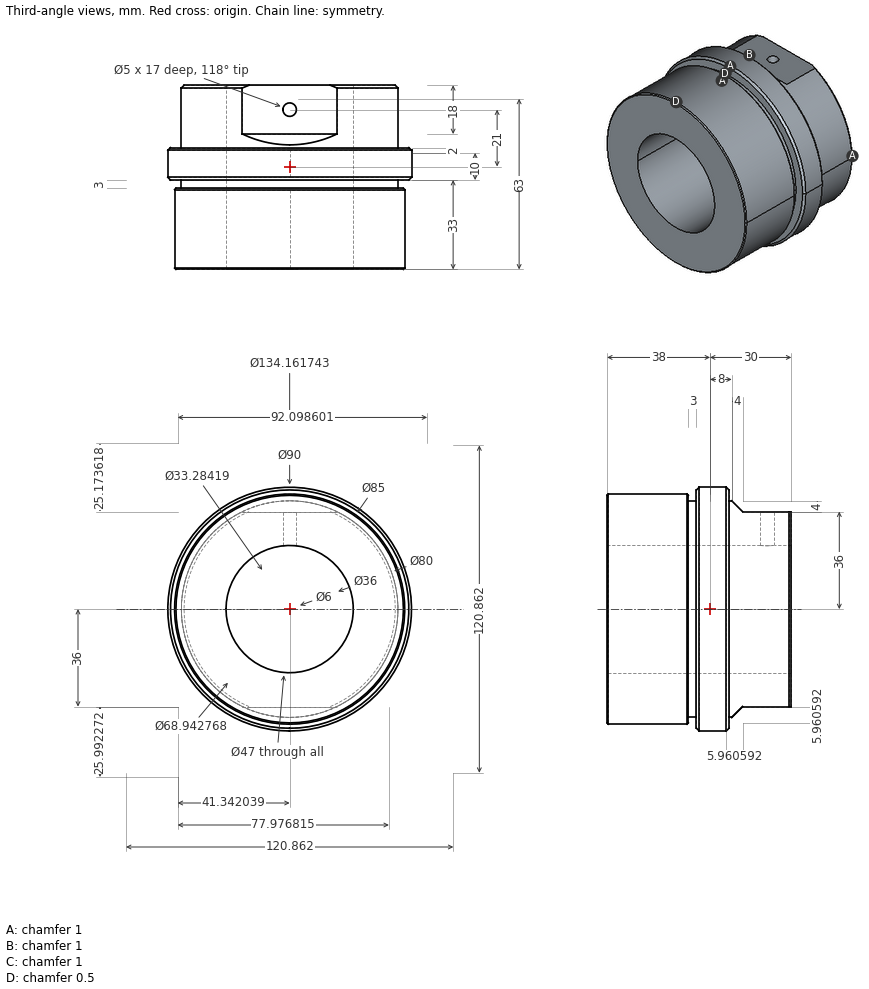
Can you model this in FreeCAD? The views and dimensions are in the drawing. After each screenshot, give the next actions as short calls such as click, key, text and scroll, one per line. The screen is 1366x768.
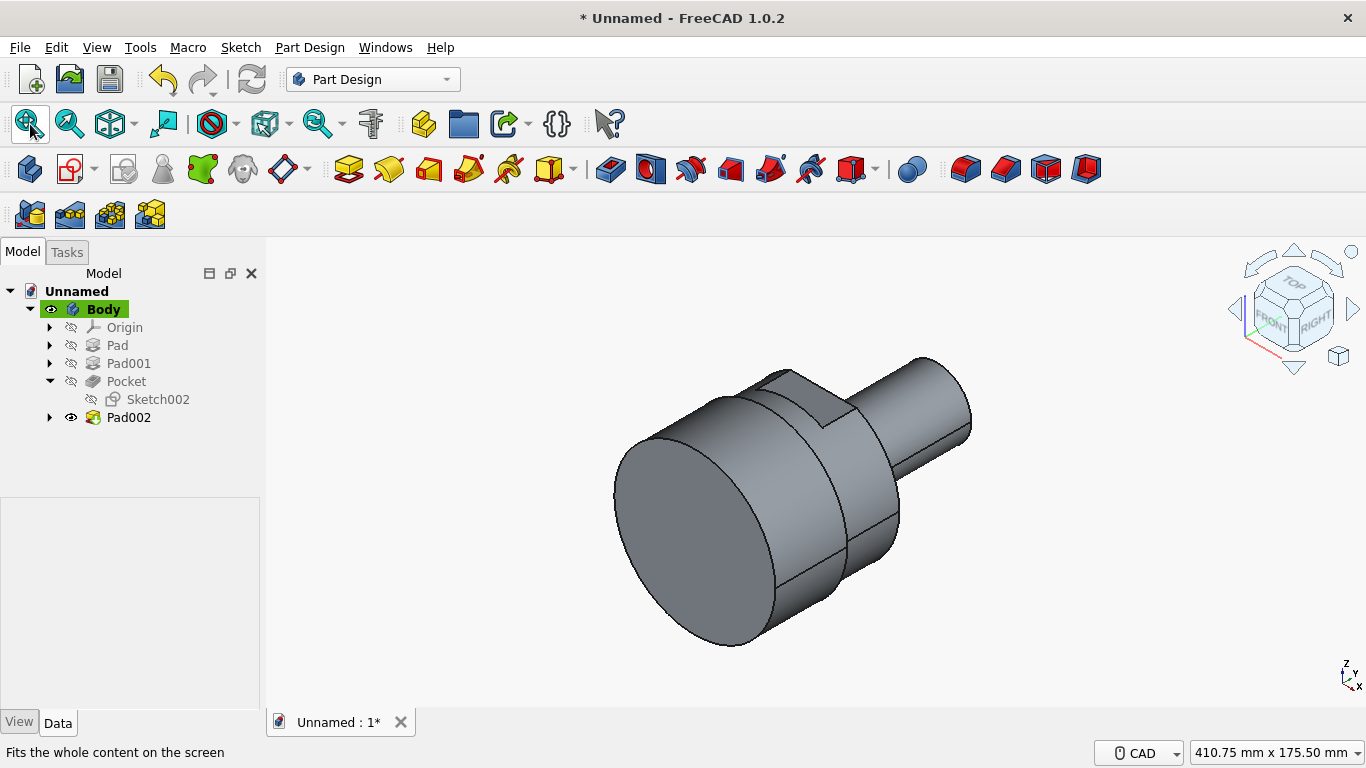
click(695, 541)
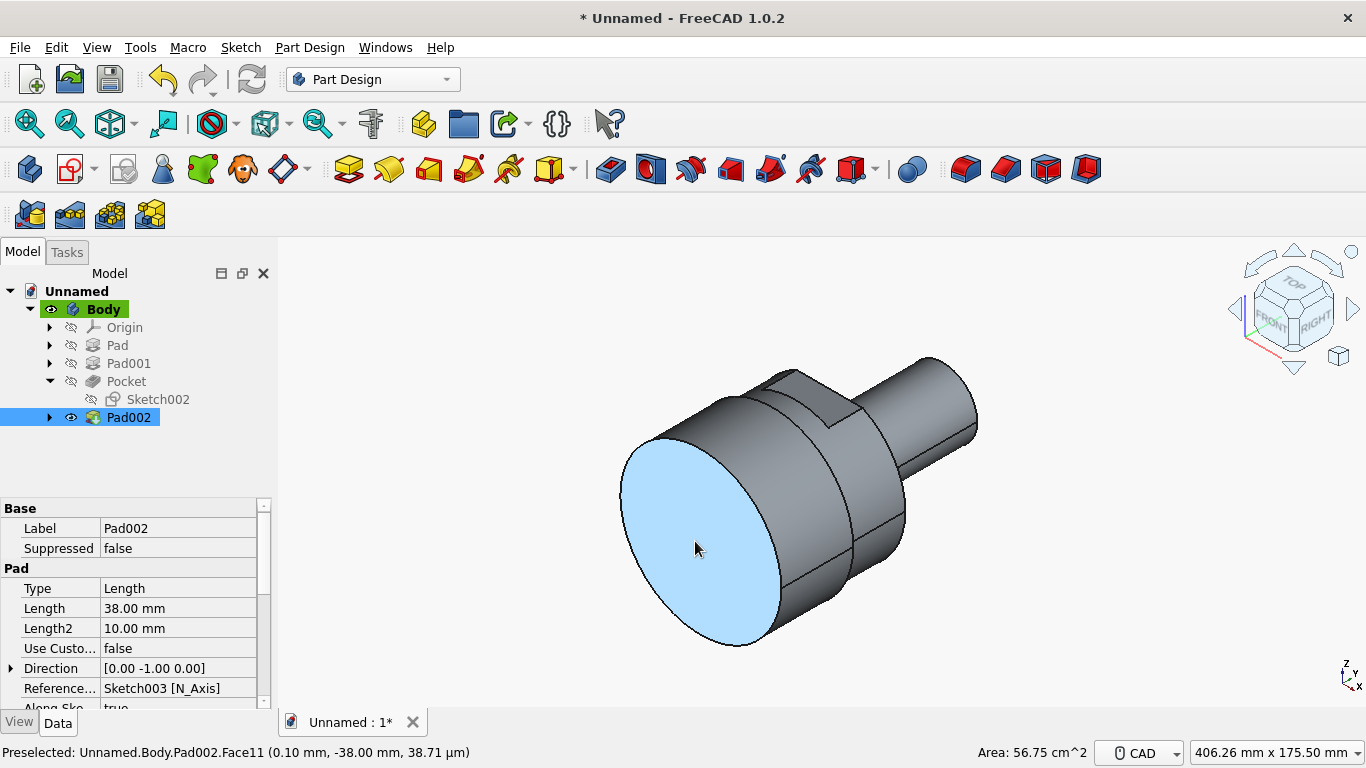
click(70, 170)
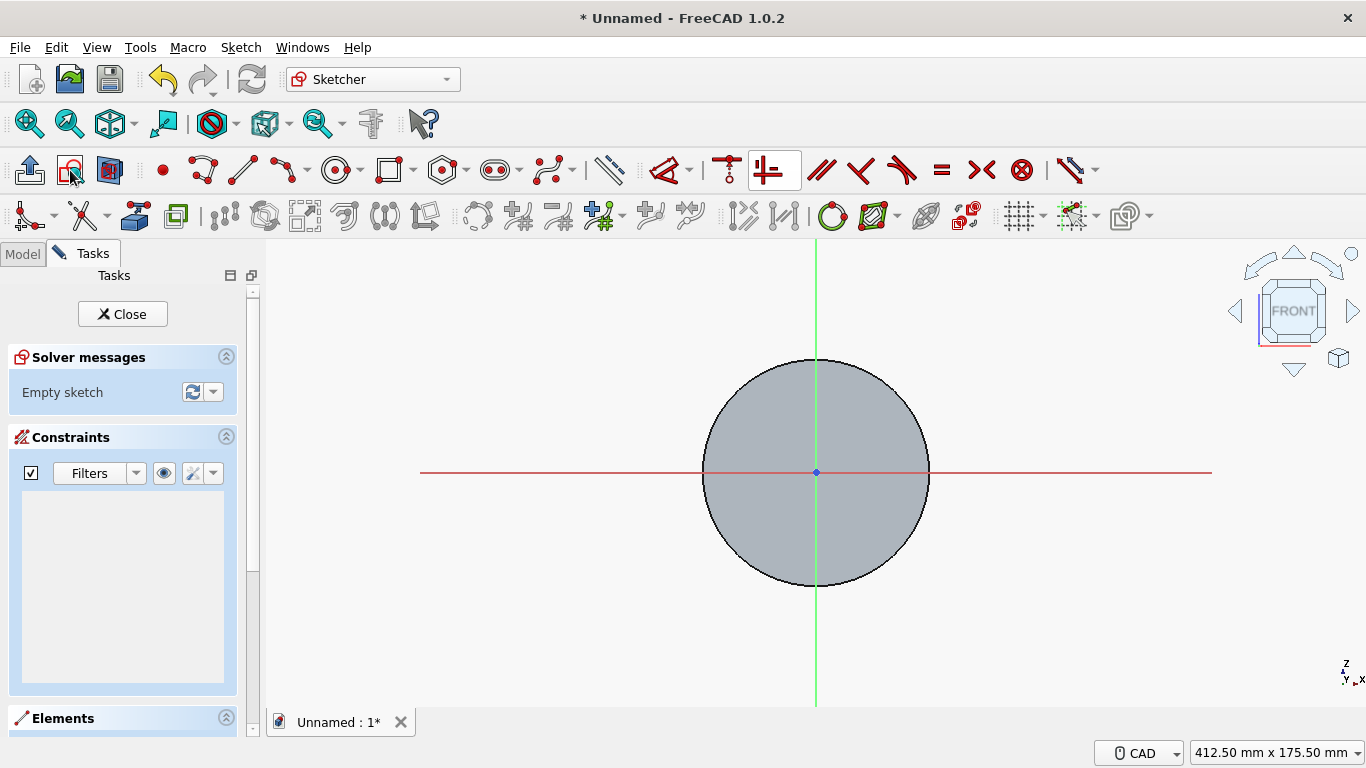
scroll(820, 473, up, 14)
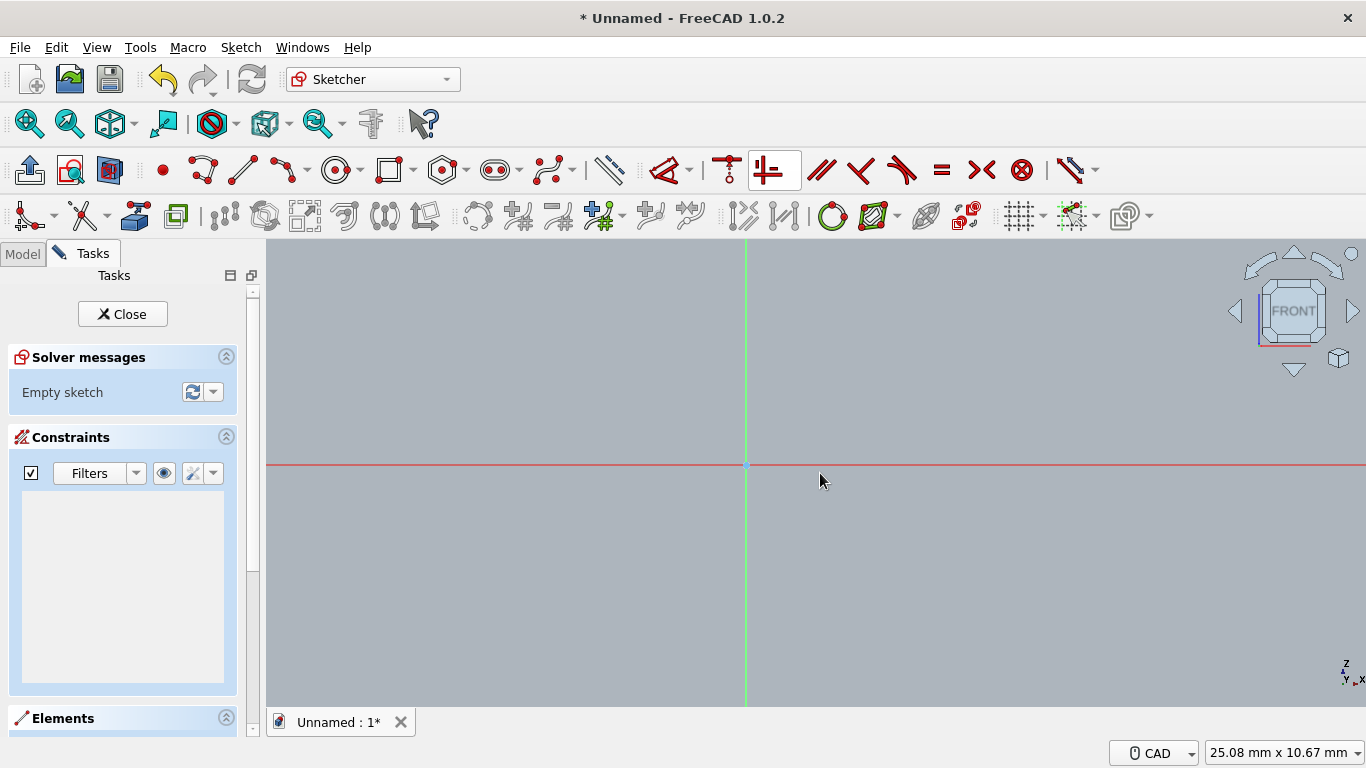
click(336, 170)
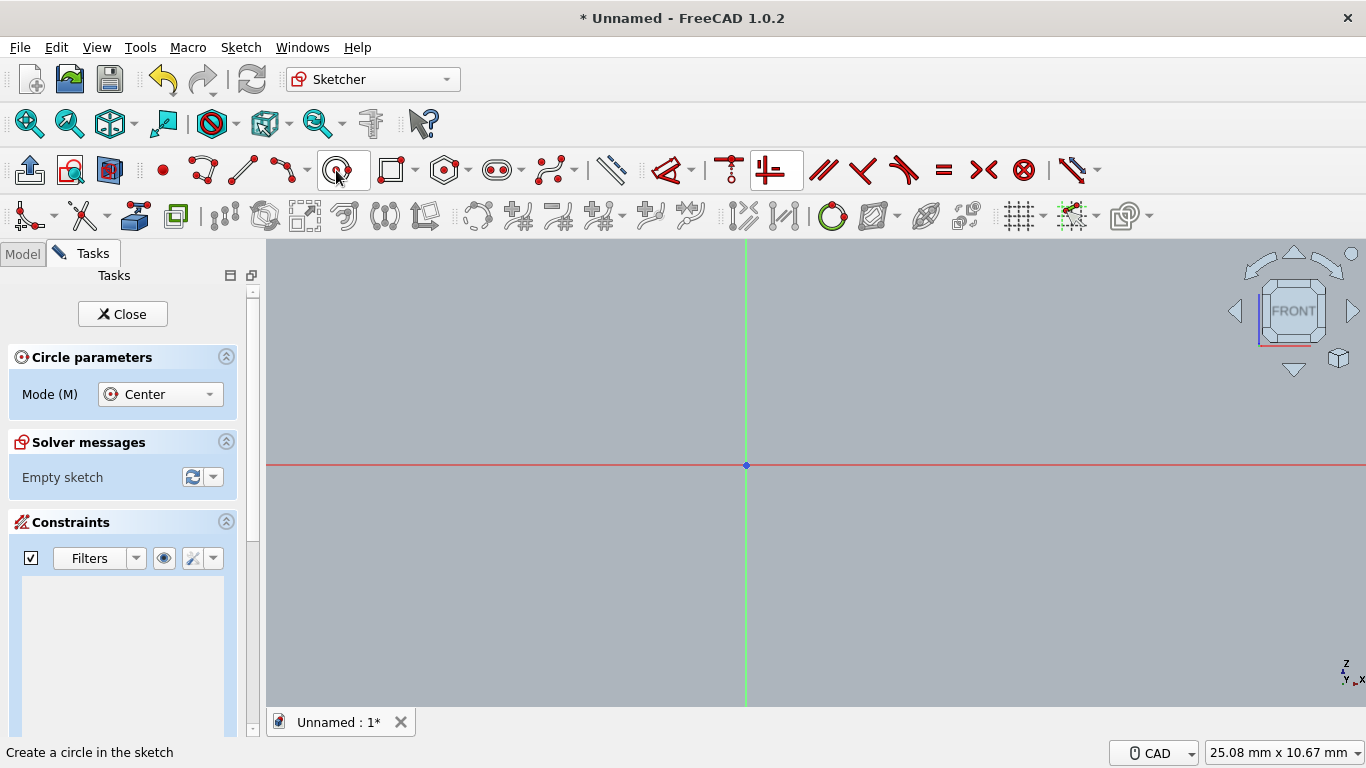
click(746, 465)
click(839, 372)
key(Escape)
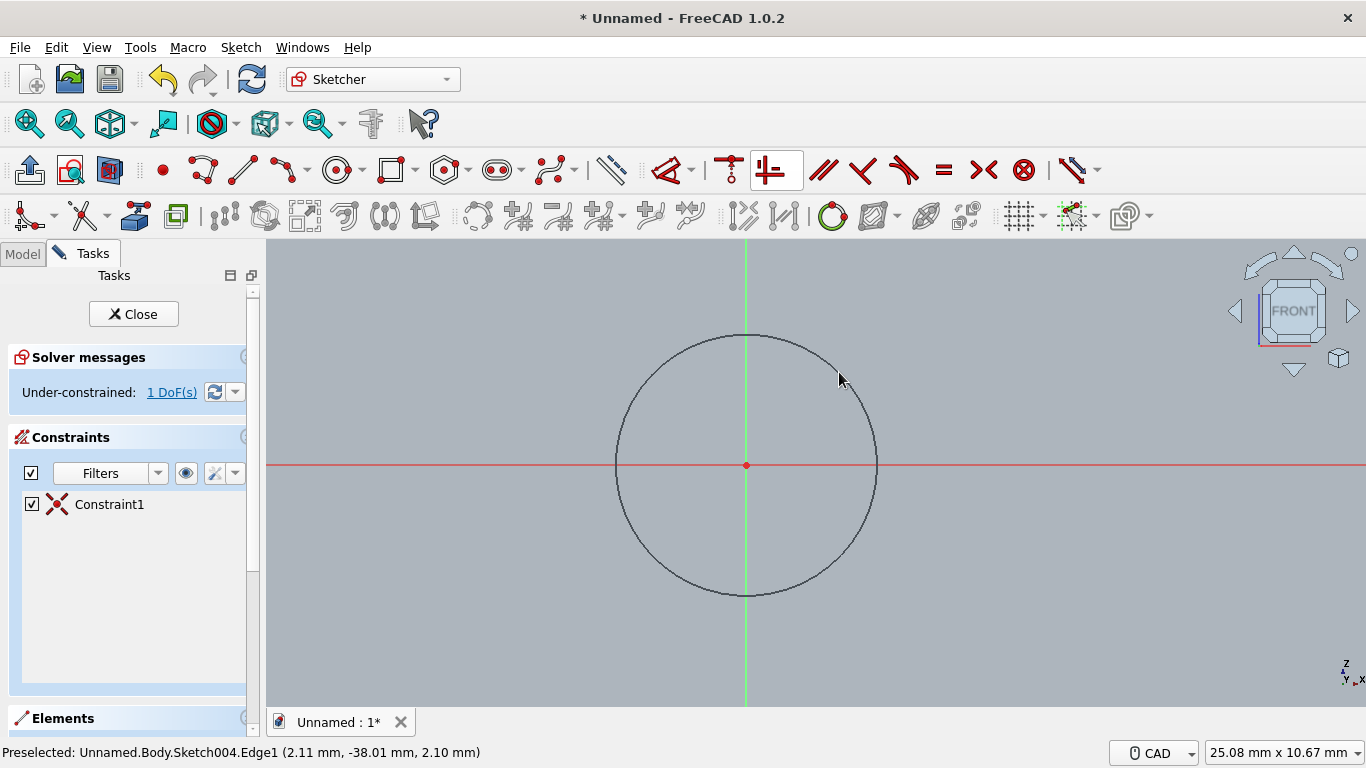
click(666, 170)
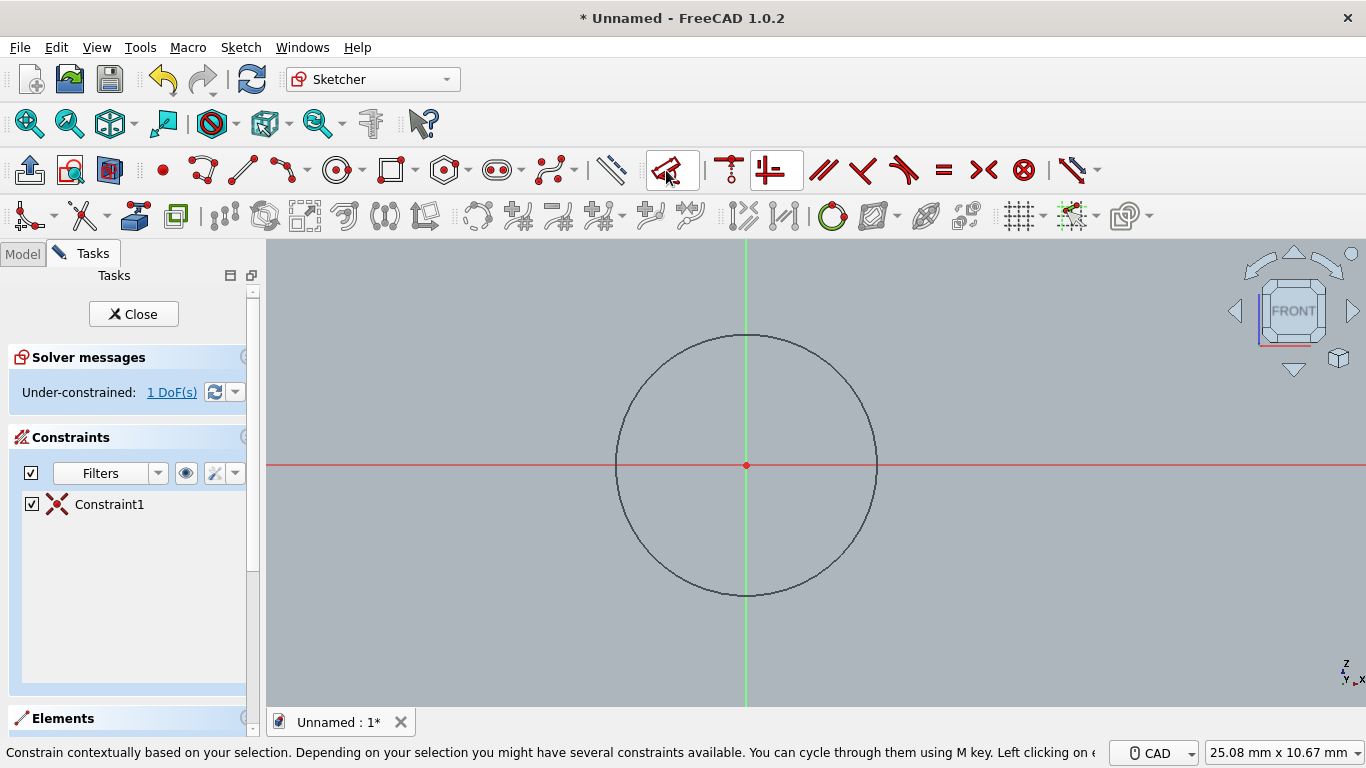
click(839, 373)
click(862, 350)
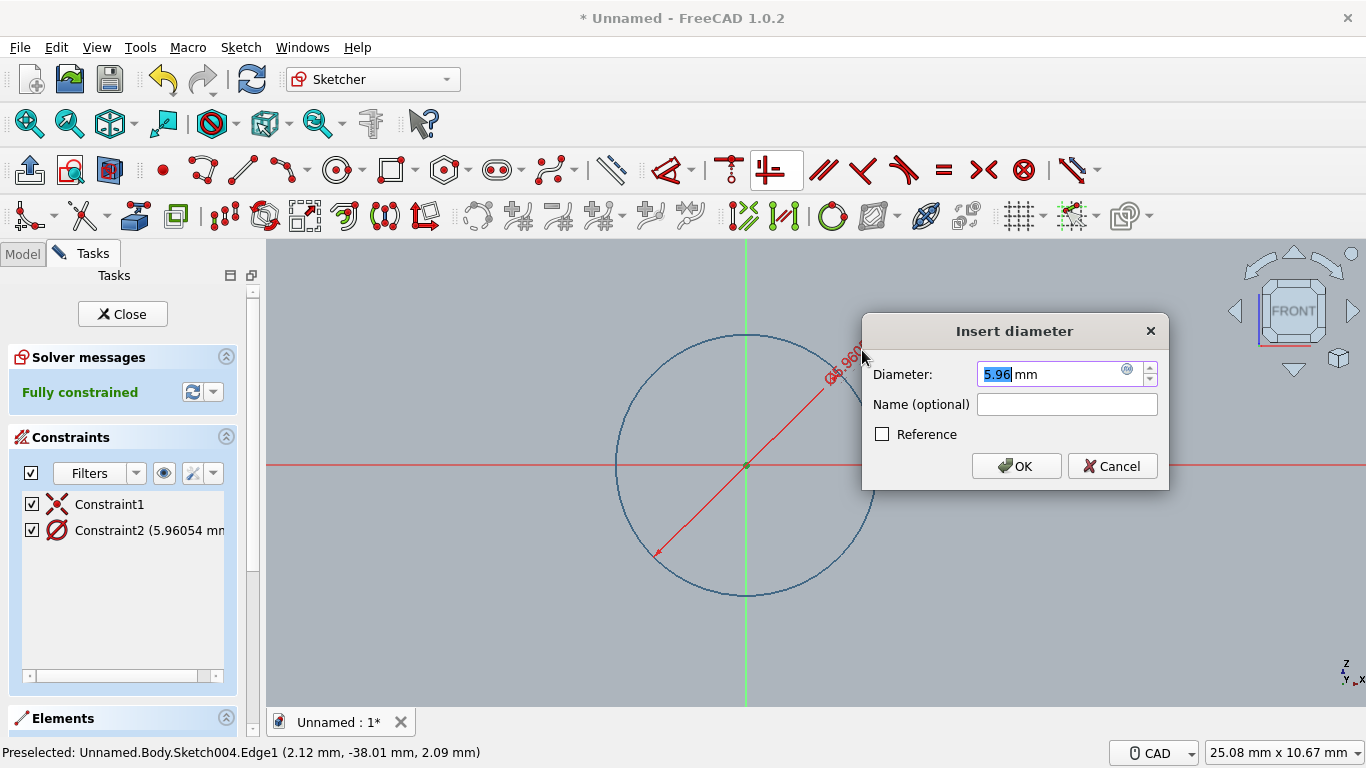
text(6)
key(Return)
key(Escape)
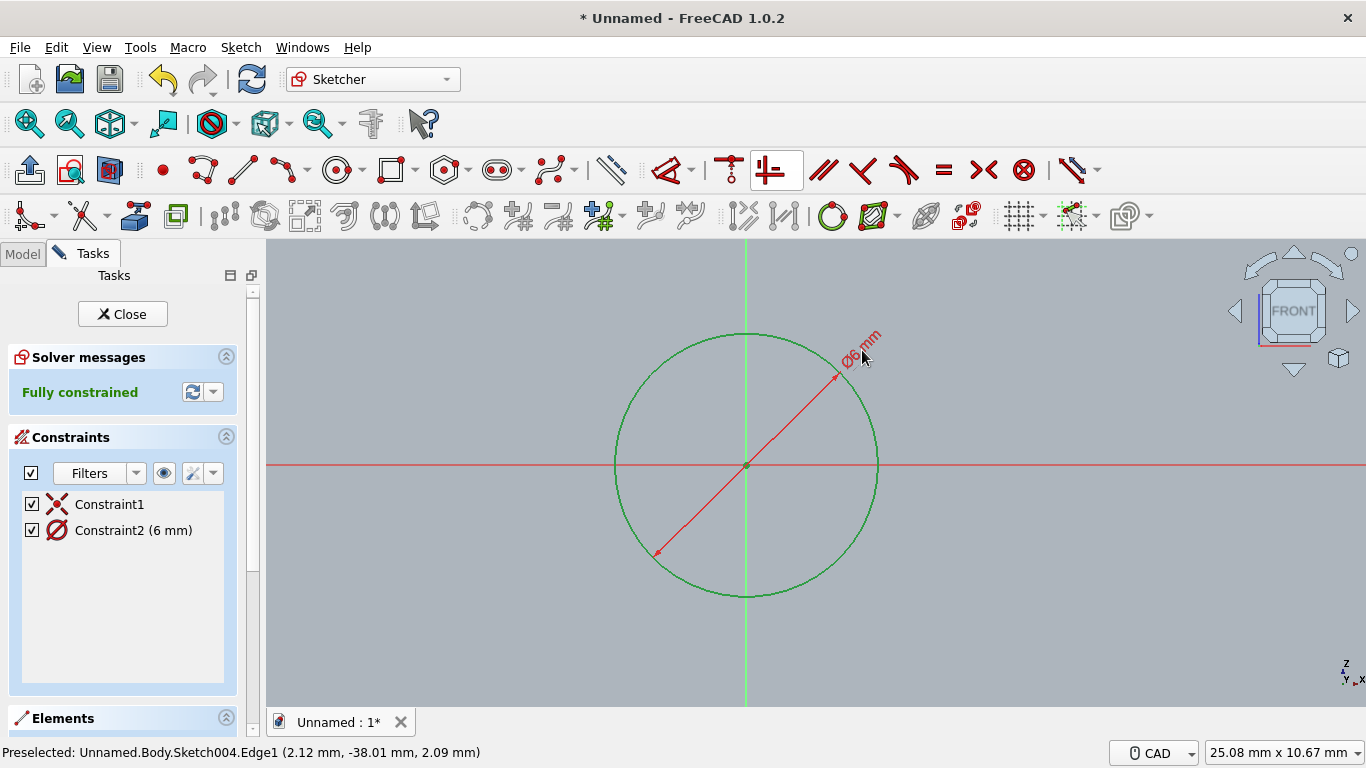
click(123, 314)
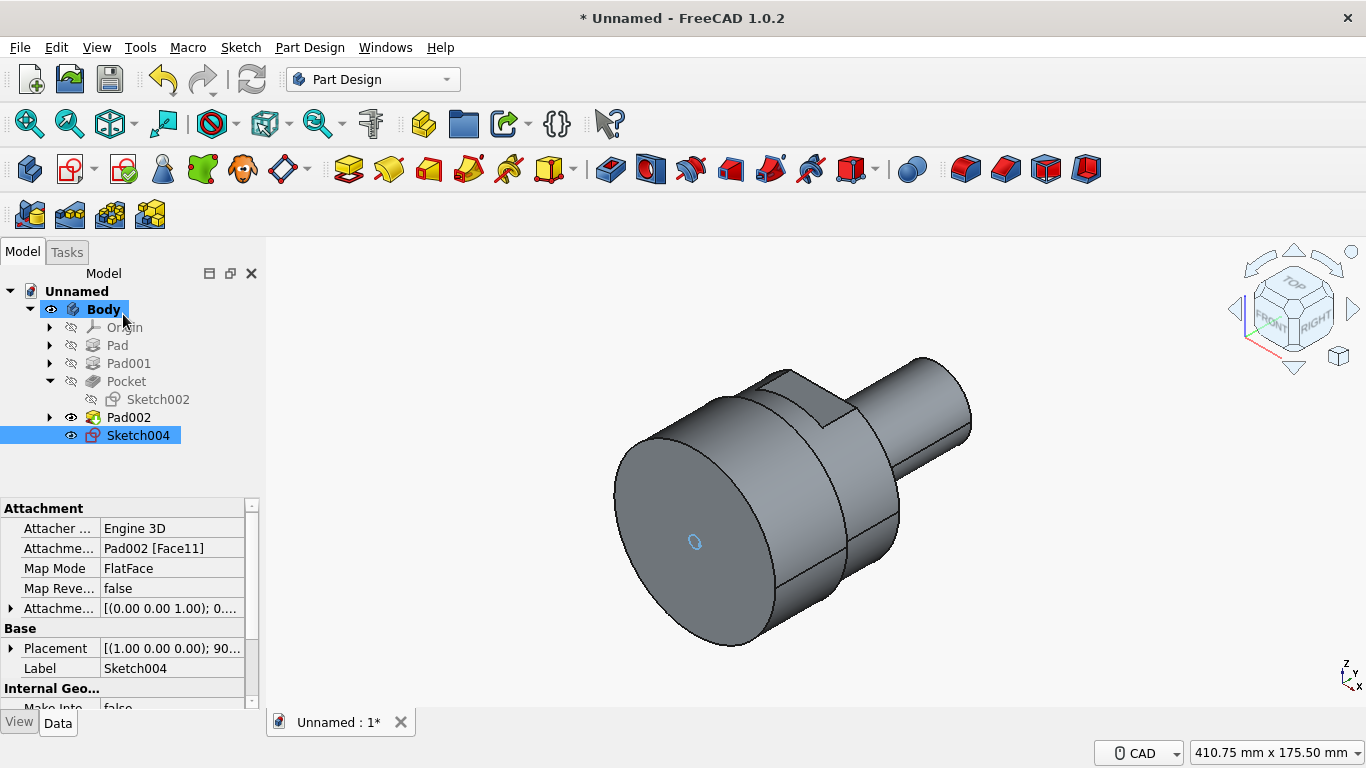
click(612, 170)